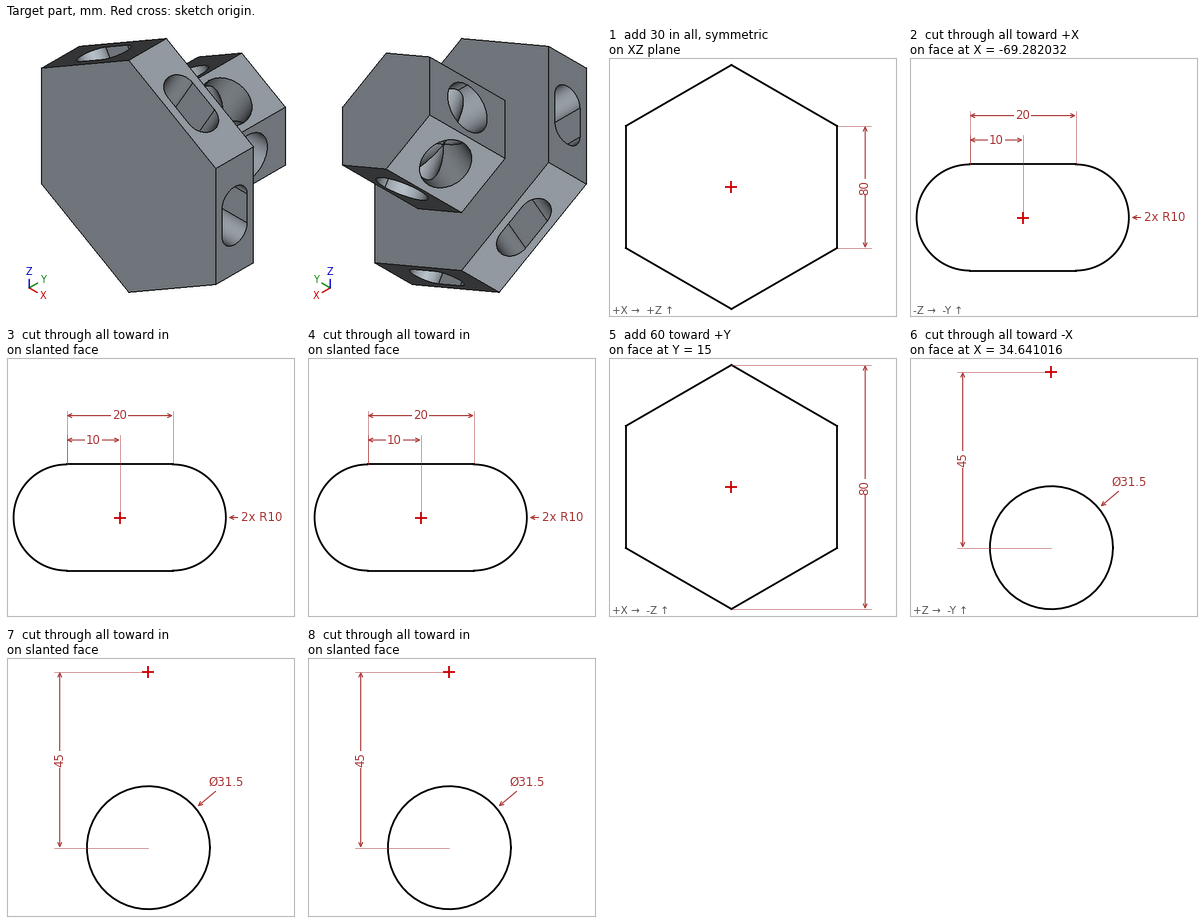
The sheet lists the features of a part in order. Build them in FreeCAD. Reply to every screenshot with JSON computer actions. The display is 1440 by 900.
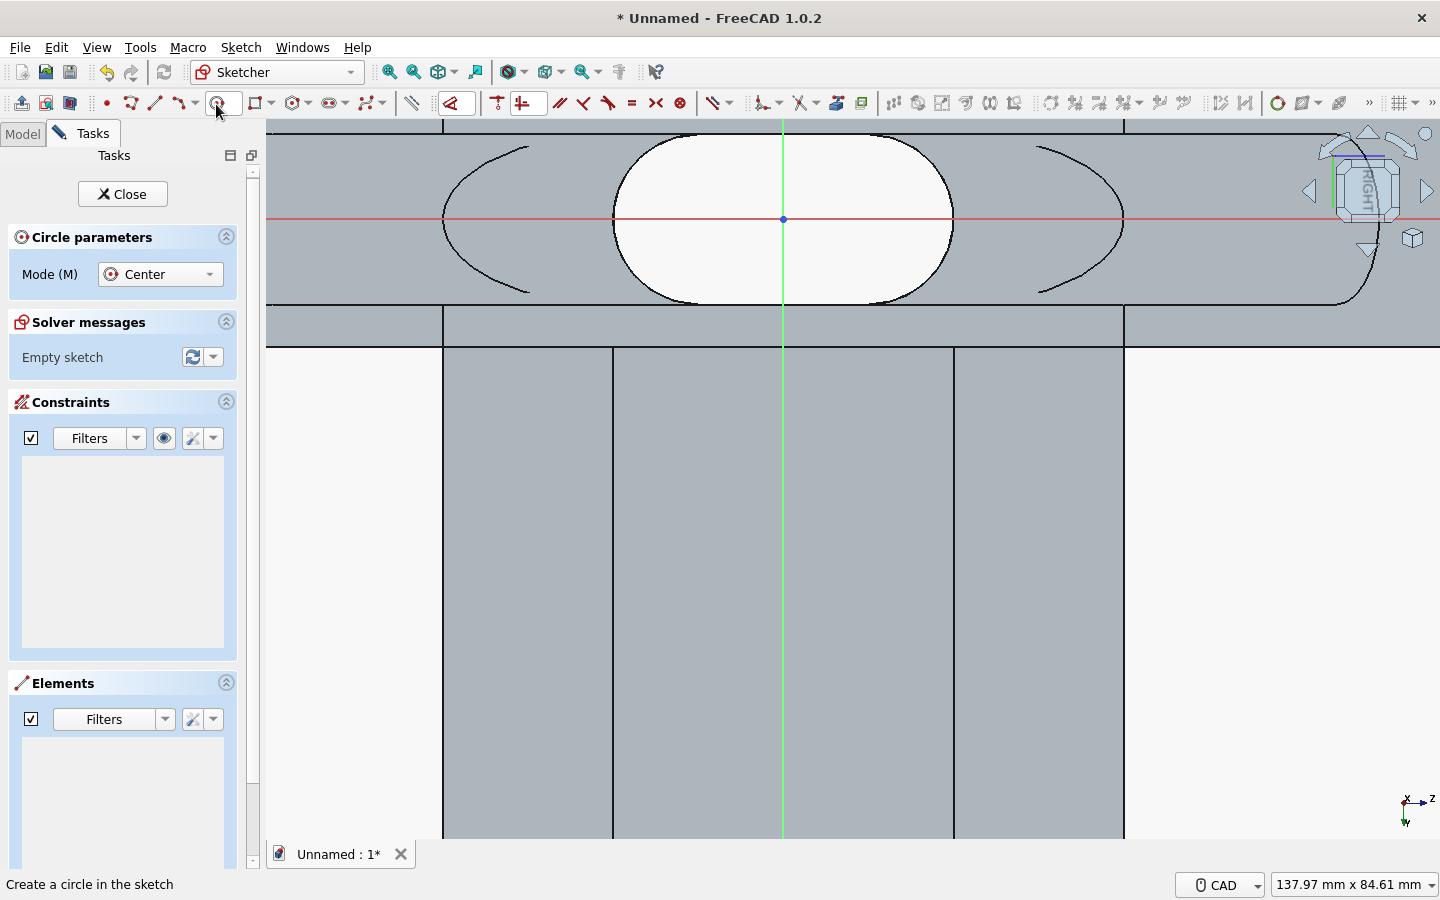
{"action": "left_click", "coordinate": [783, 602]}
{"action": "mouse_move", "coordinate": [878, 508]}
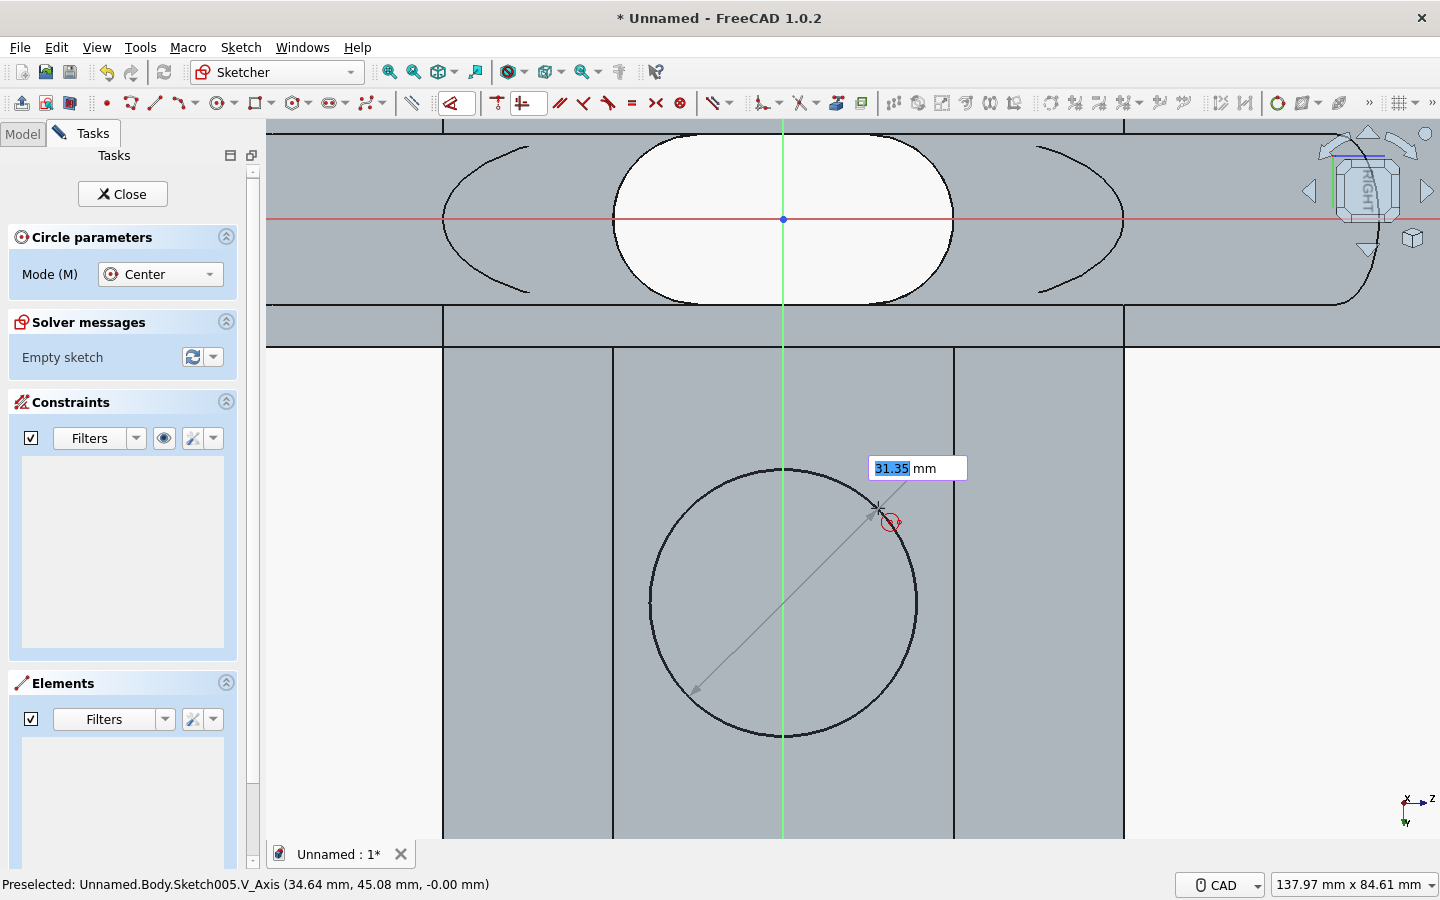
{"action": "type", "text": "31.5"}
{"action": "key", "text": "Return"}
{"action": "key", "text": "Escape"}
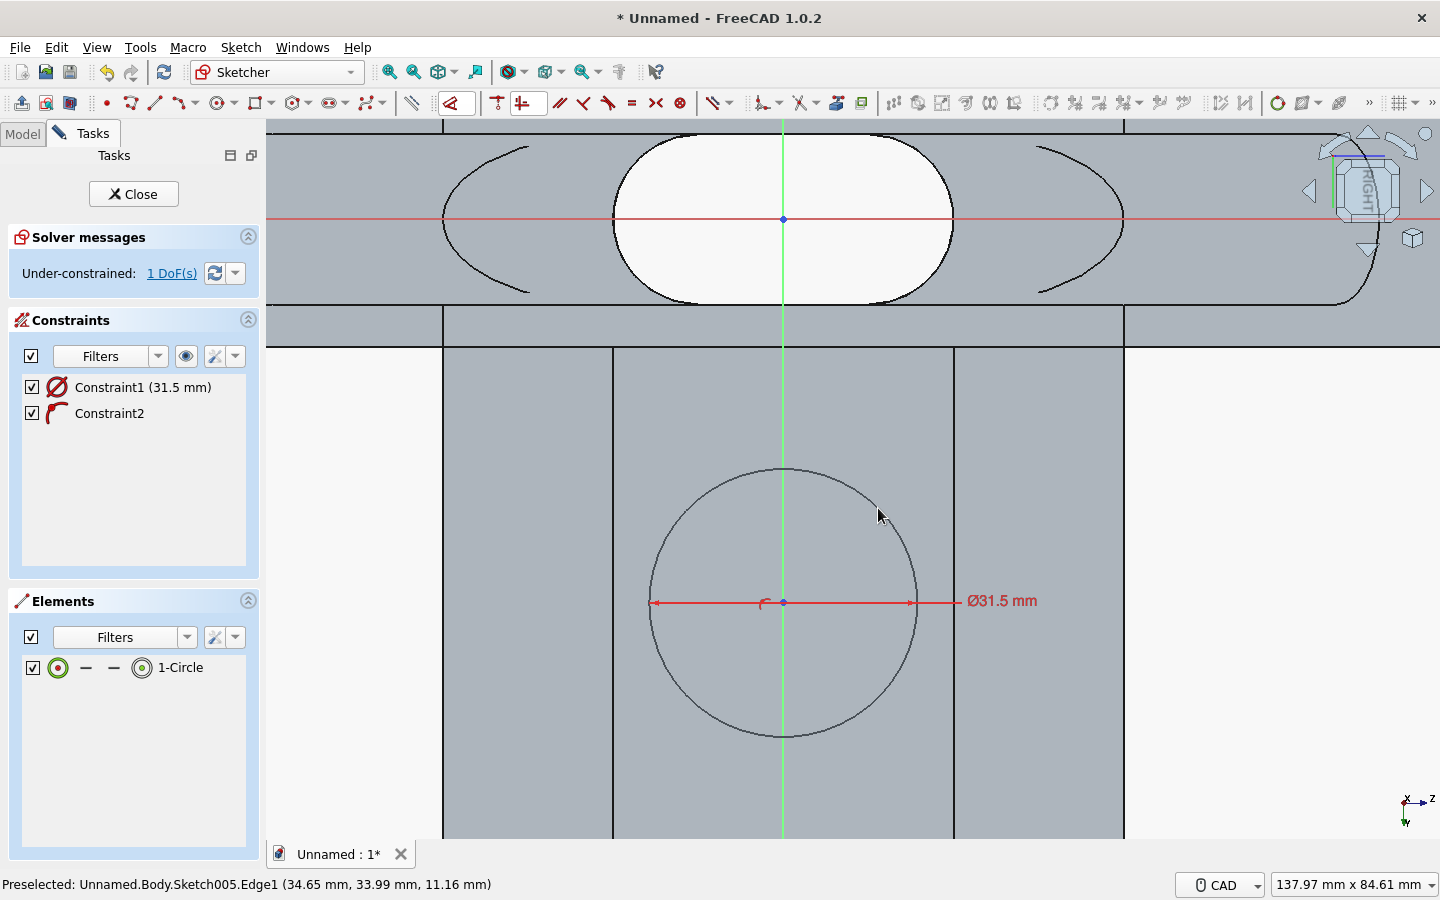
{"action": "left_click", "coordinate": [783, 603]}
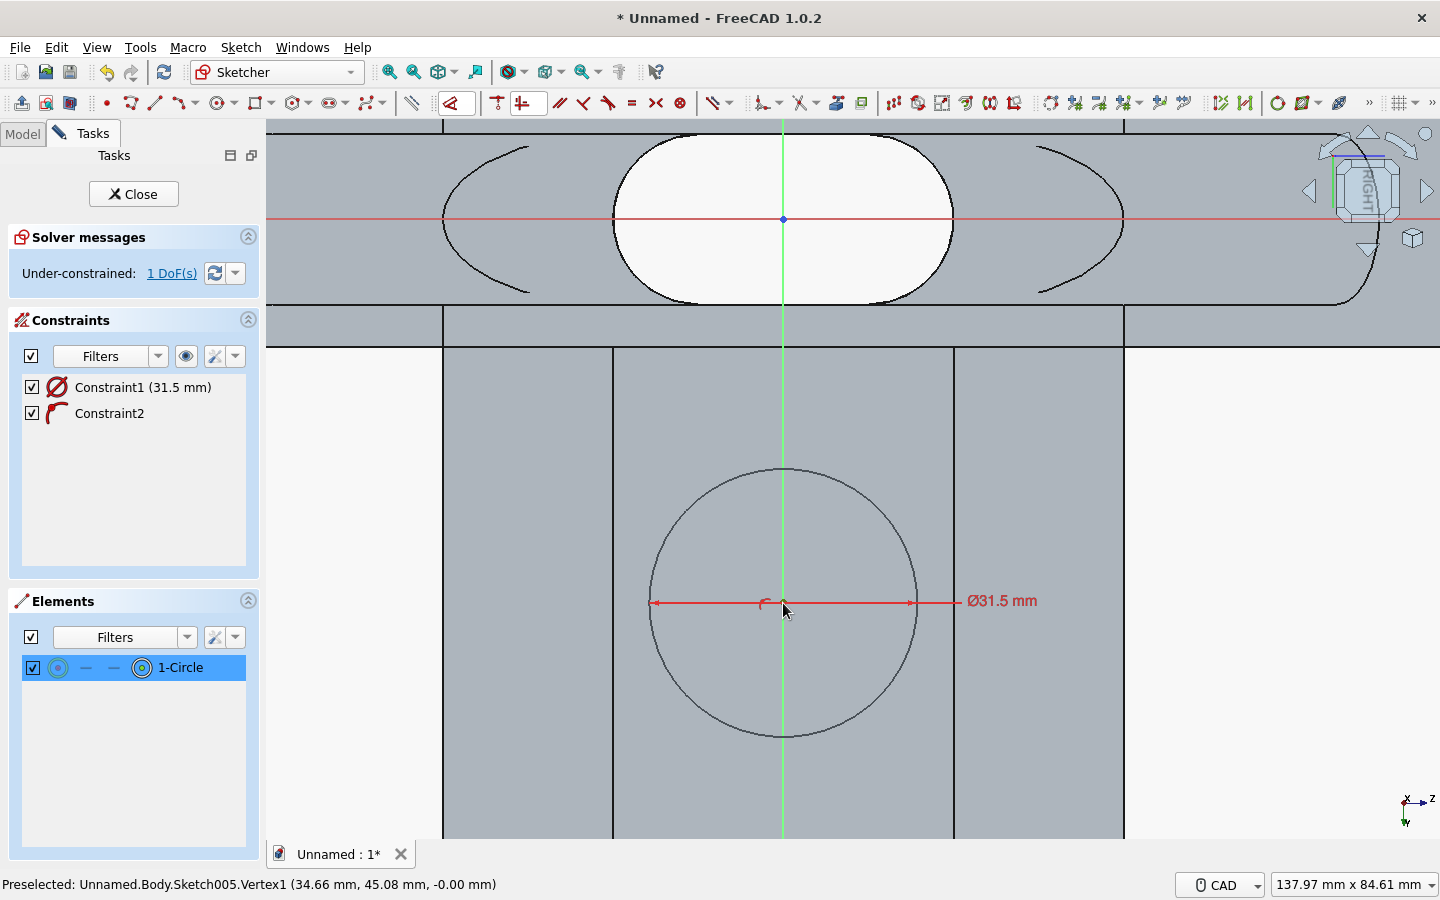
{"action": "left_click", "coordinate": [470, 104]}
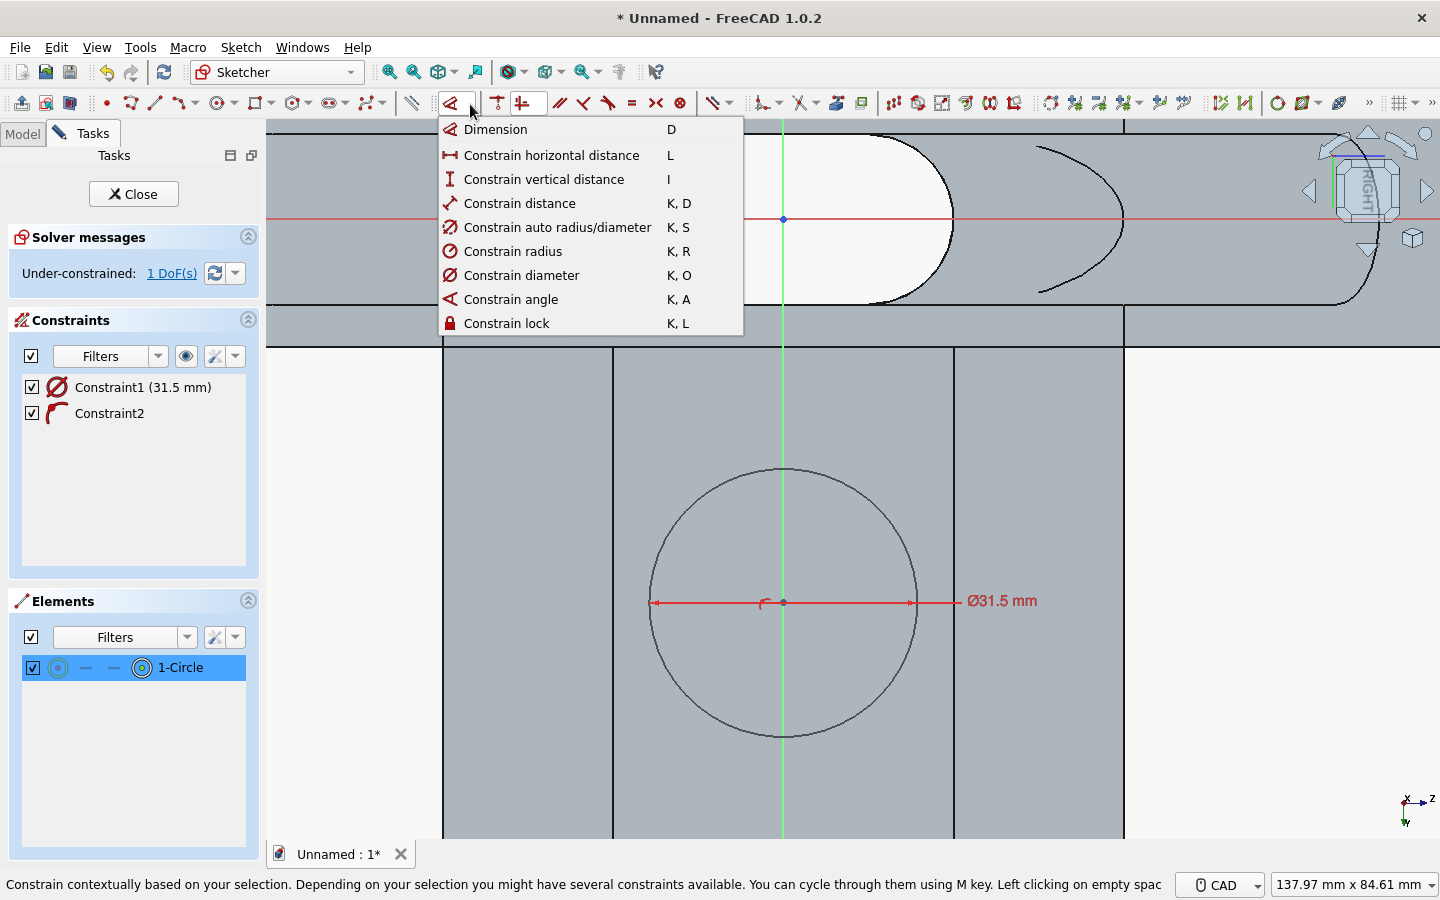
{"action": "left_click", "coordinate": [591, 179]}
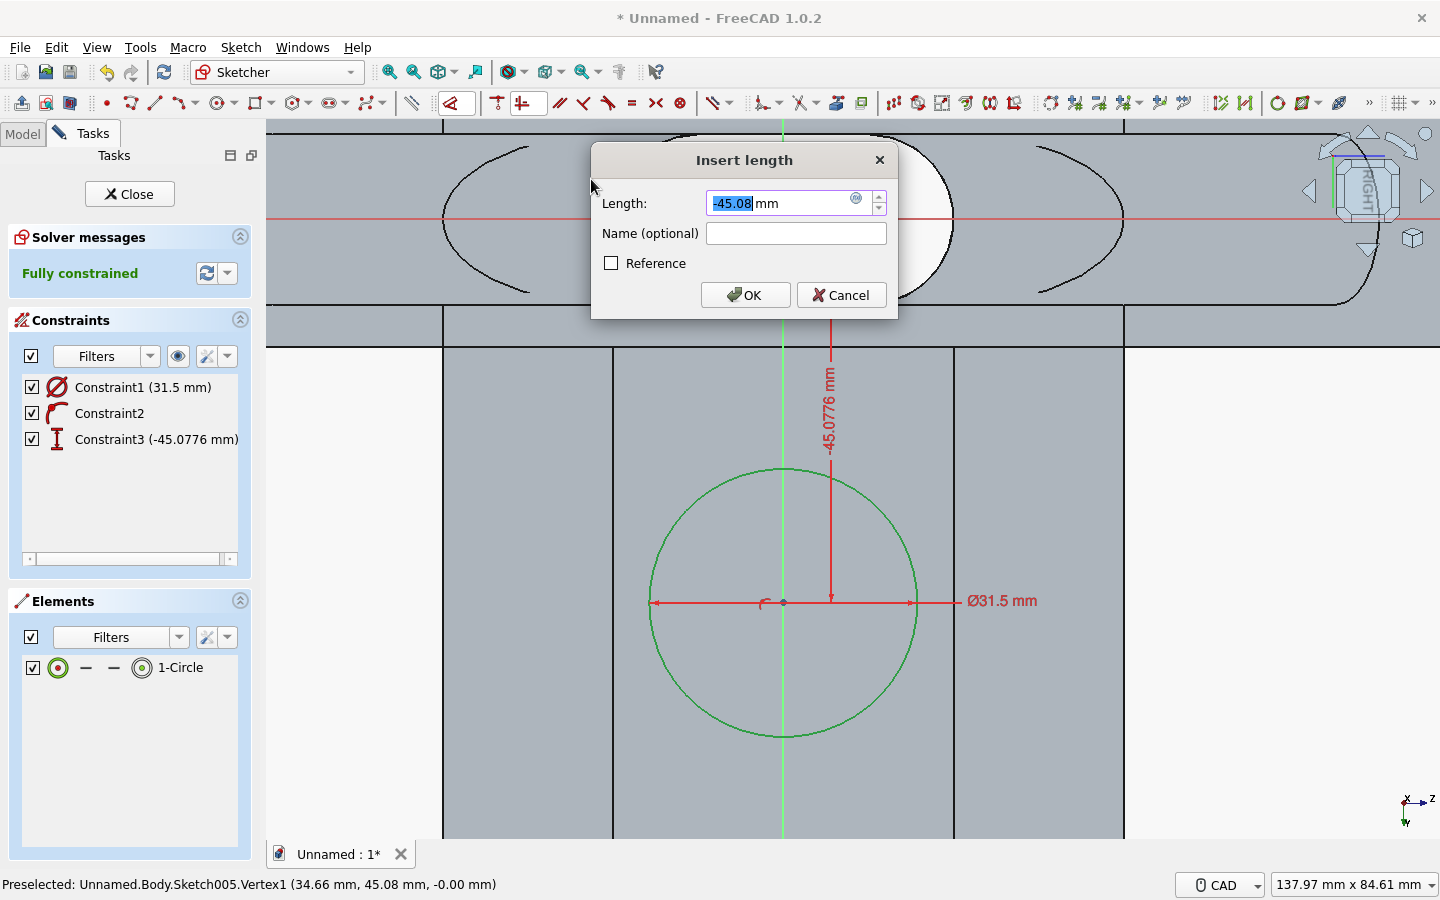
{"action": "type", "text": "-45"}
{"action": "key", "text": "Return"}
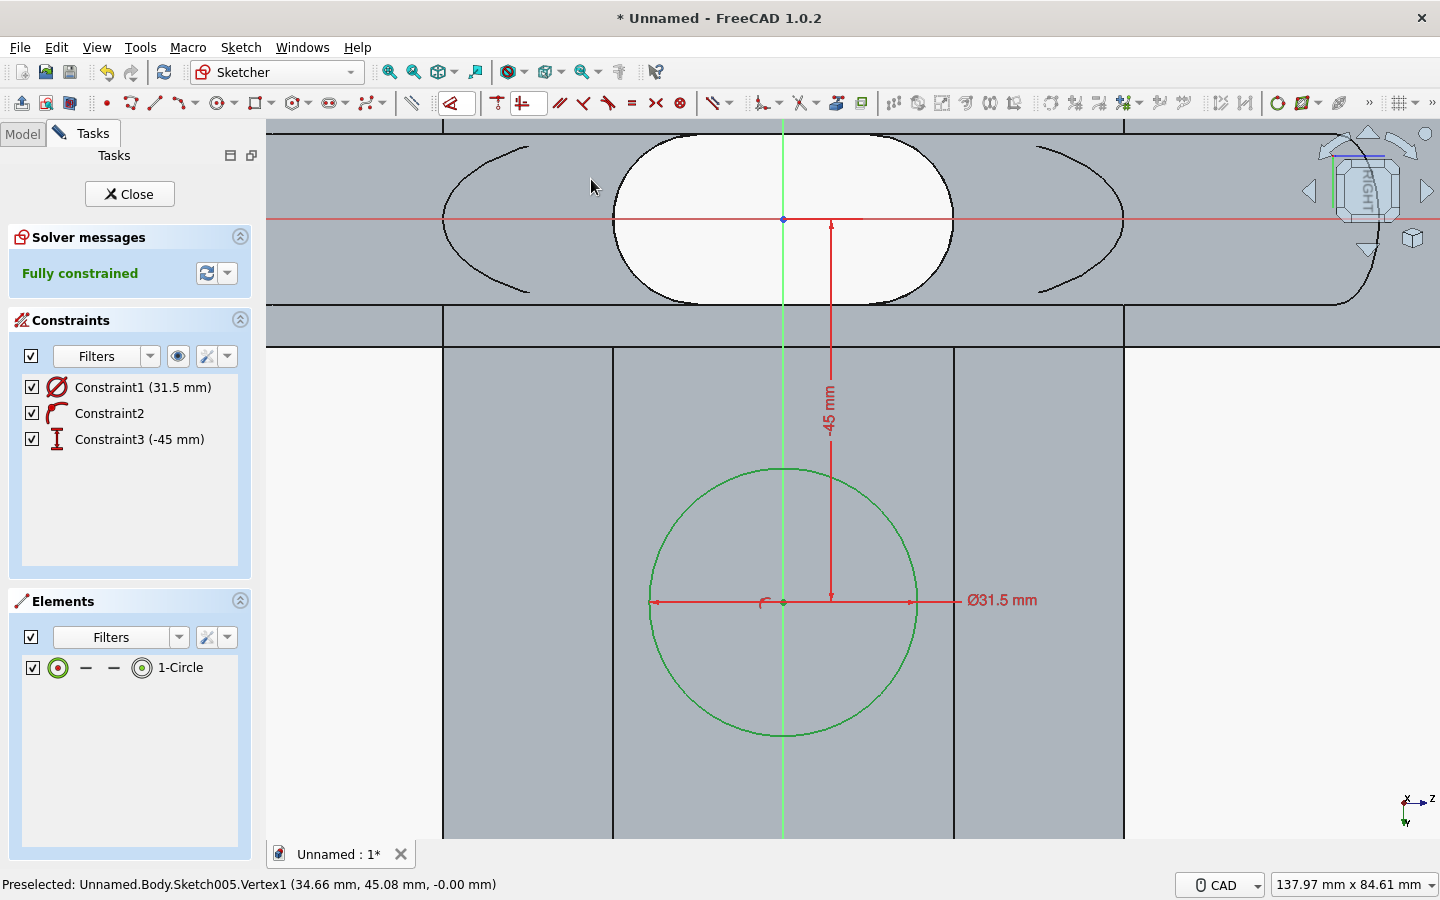
{"action": "left_click", "coordinate": [130, 194]}